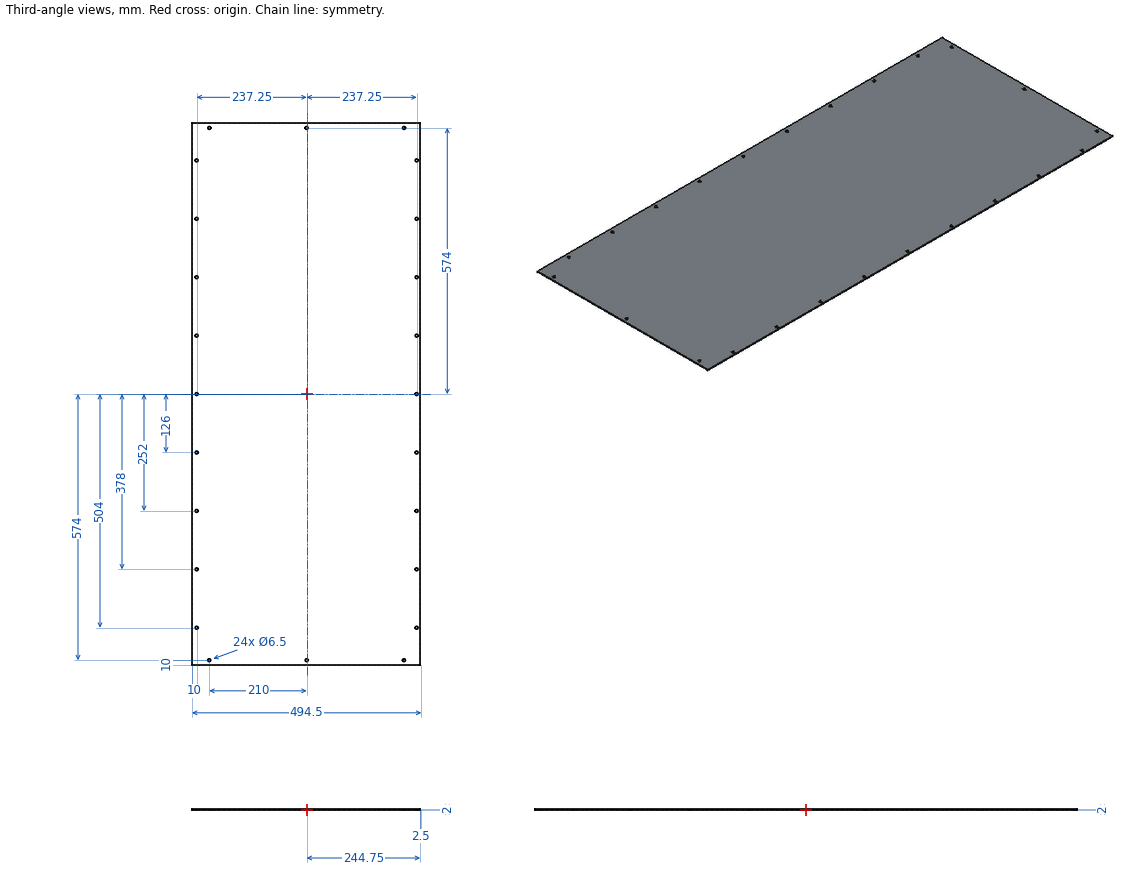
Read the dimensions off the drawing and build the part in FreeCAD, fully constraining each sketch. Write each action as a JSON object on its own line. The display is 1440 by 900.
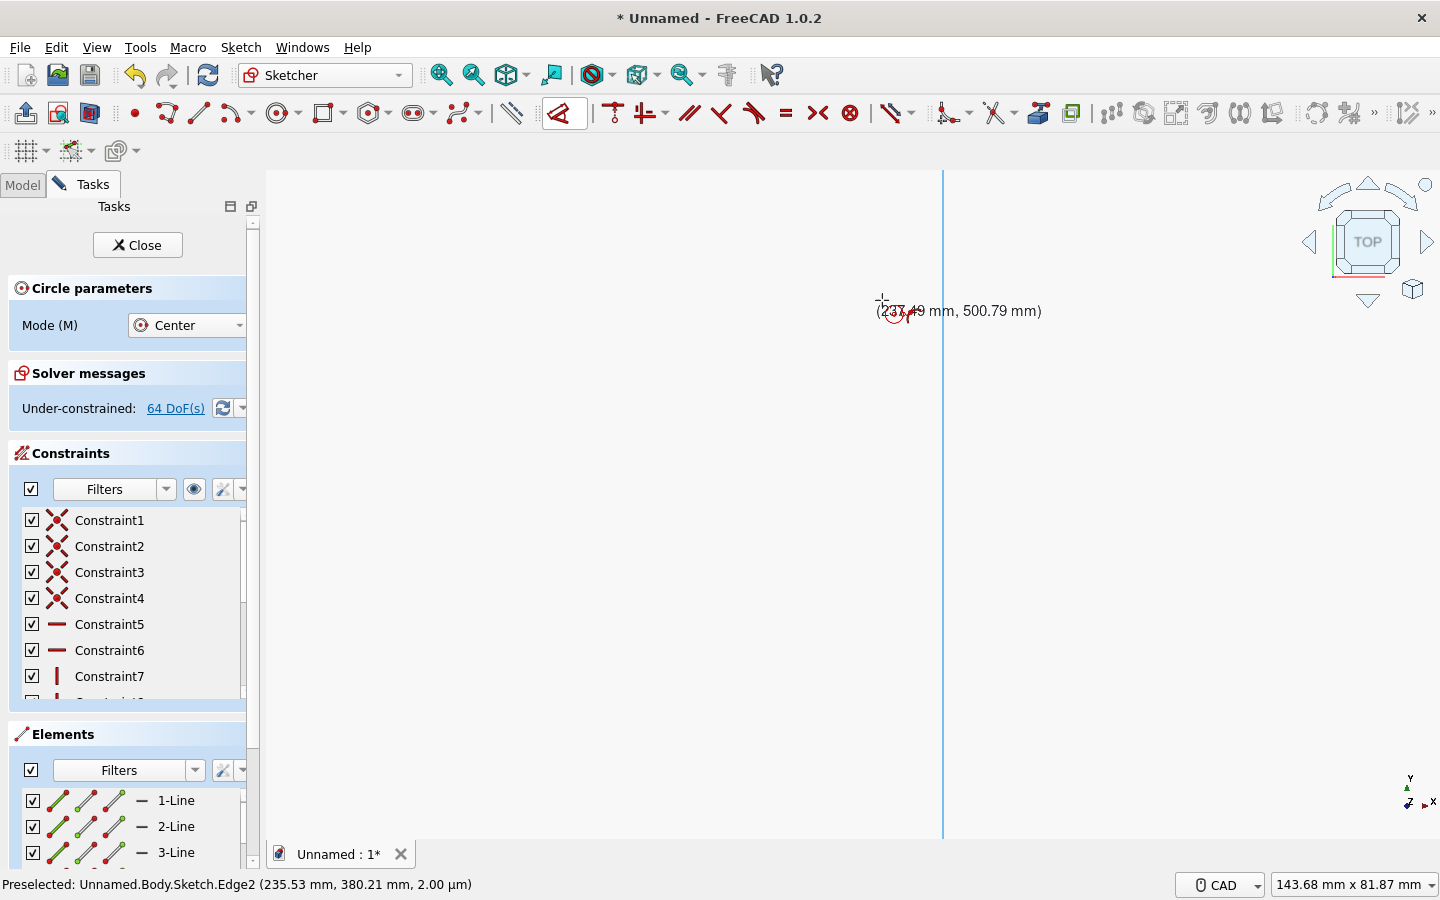
{"action": "scroll", "coordinate": [882, 300], "scroll_direction": "down", "scroll_amount": 15}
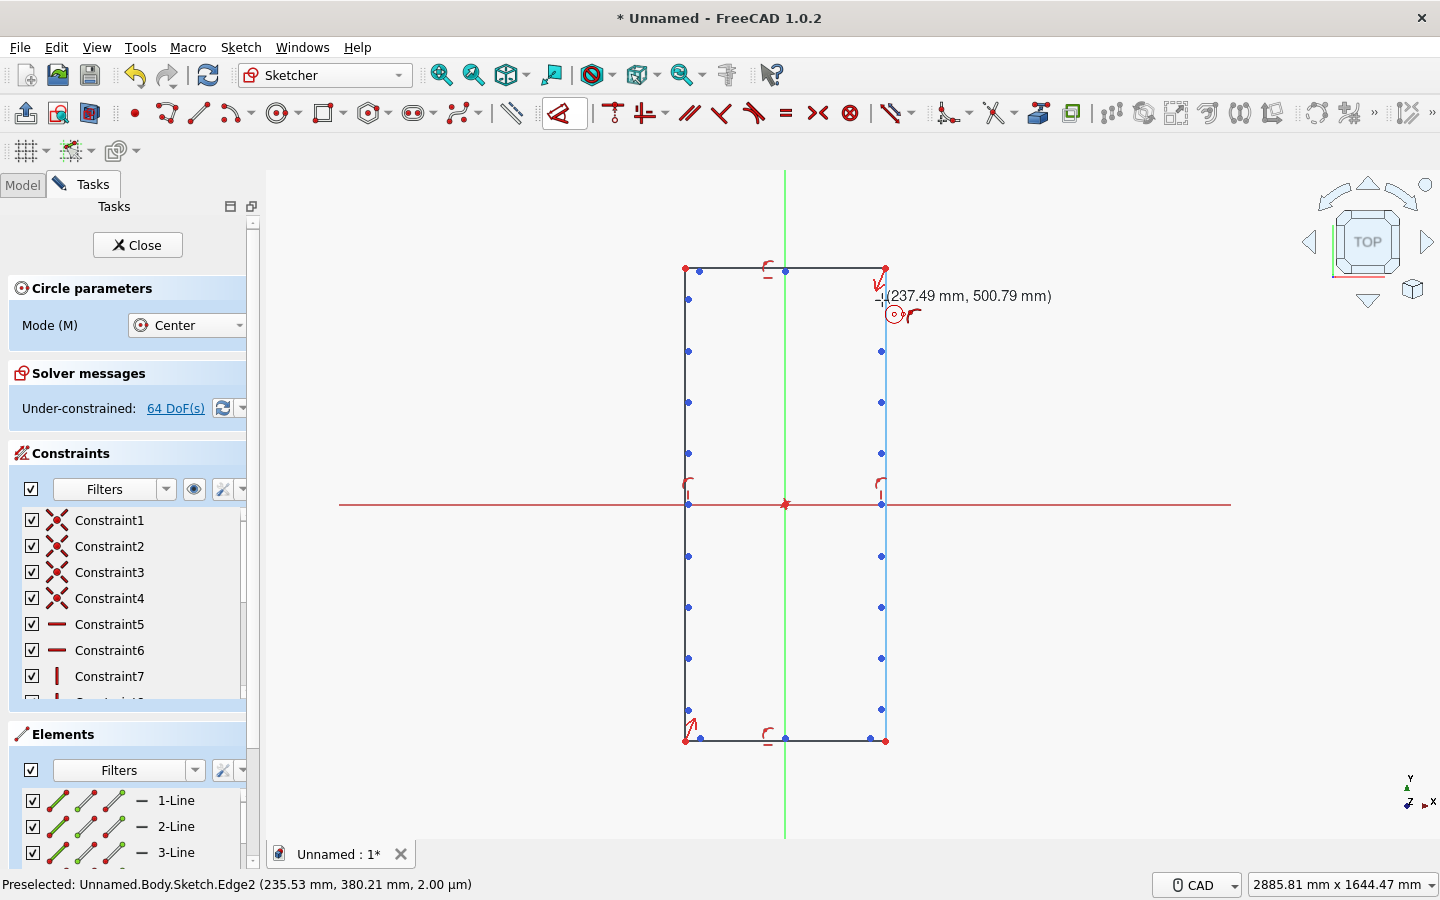
{"action": "scroll", "coordinate": [882, 300], "scroll_direction": "up", "scroll_amount": 7}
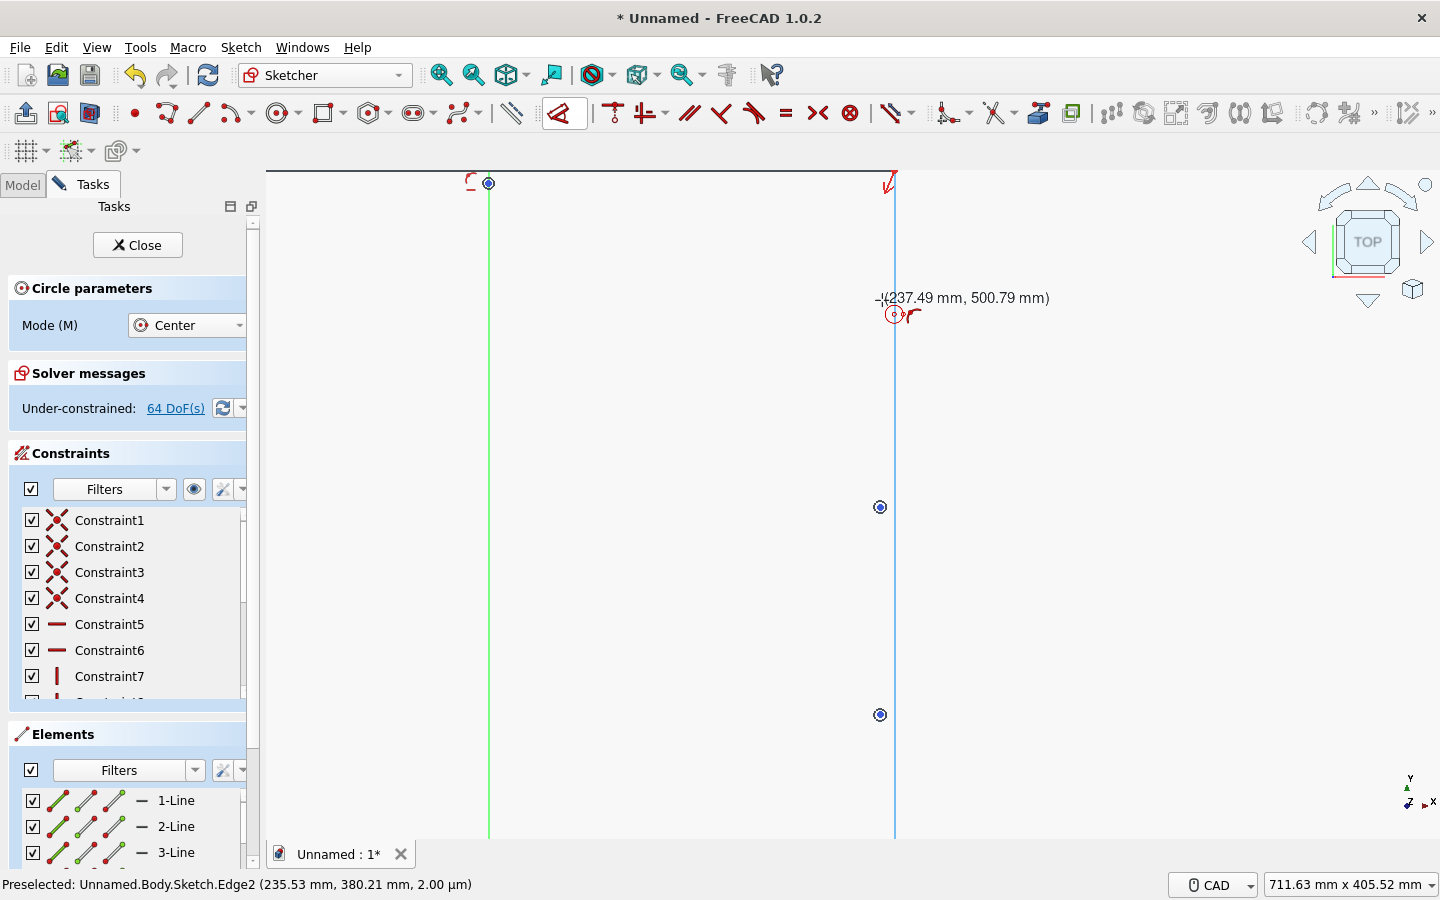
{"action": "left_click", "coordinate": [880, 298]}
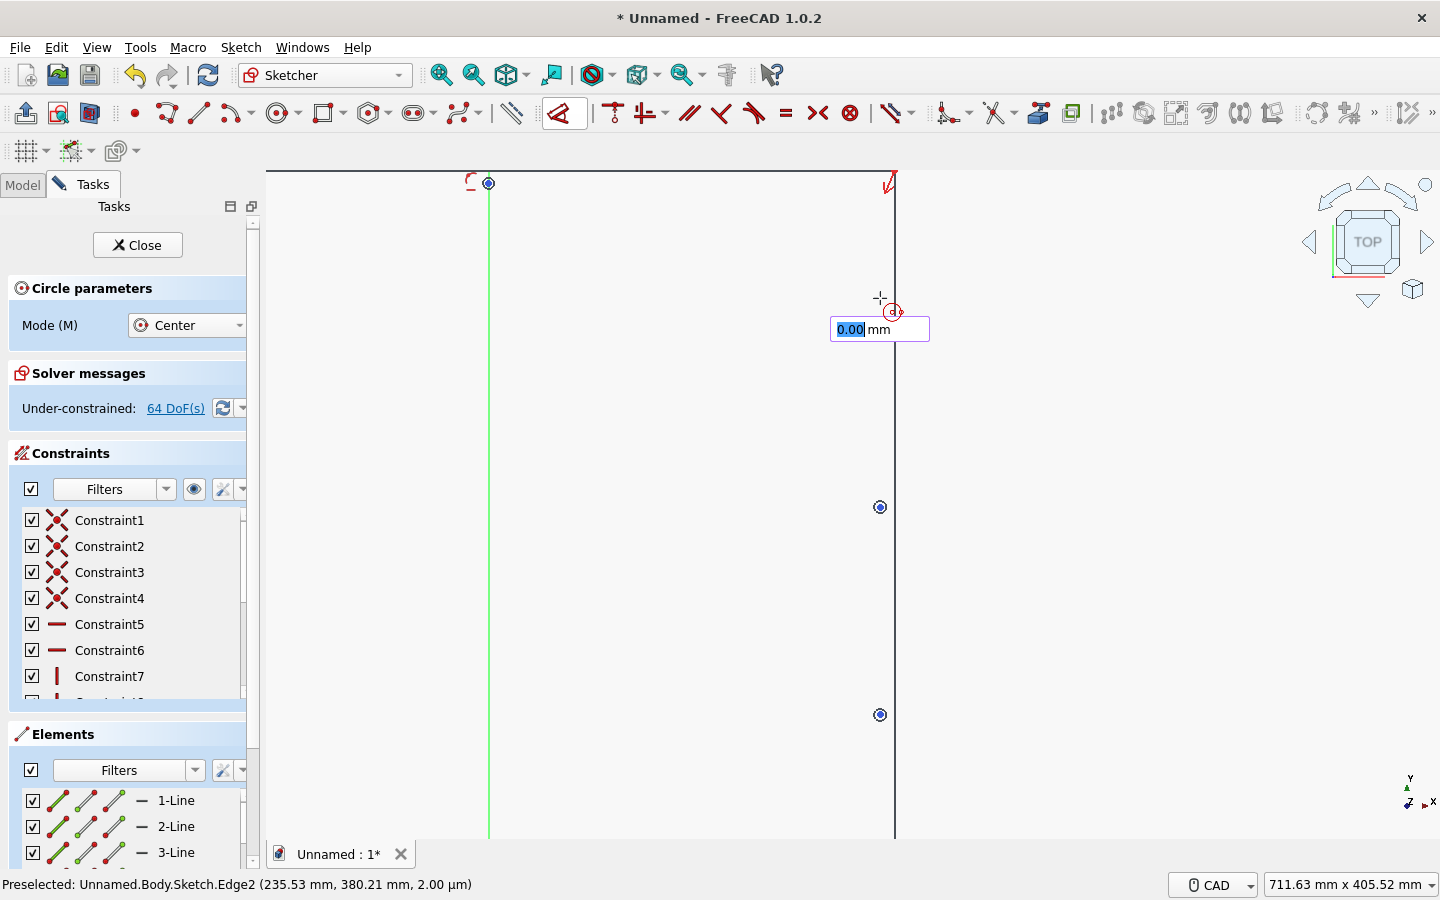
{"action": "scroll", "coordinate": [876, 294], "scroll_direction": "up", "scroll_amount": 6}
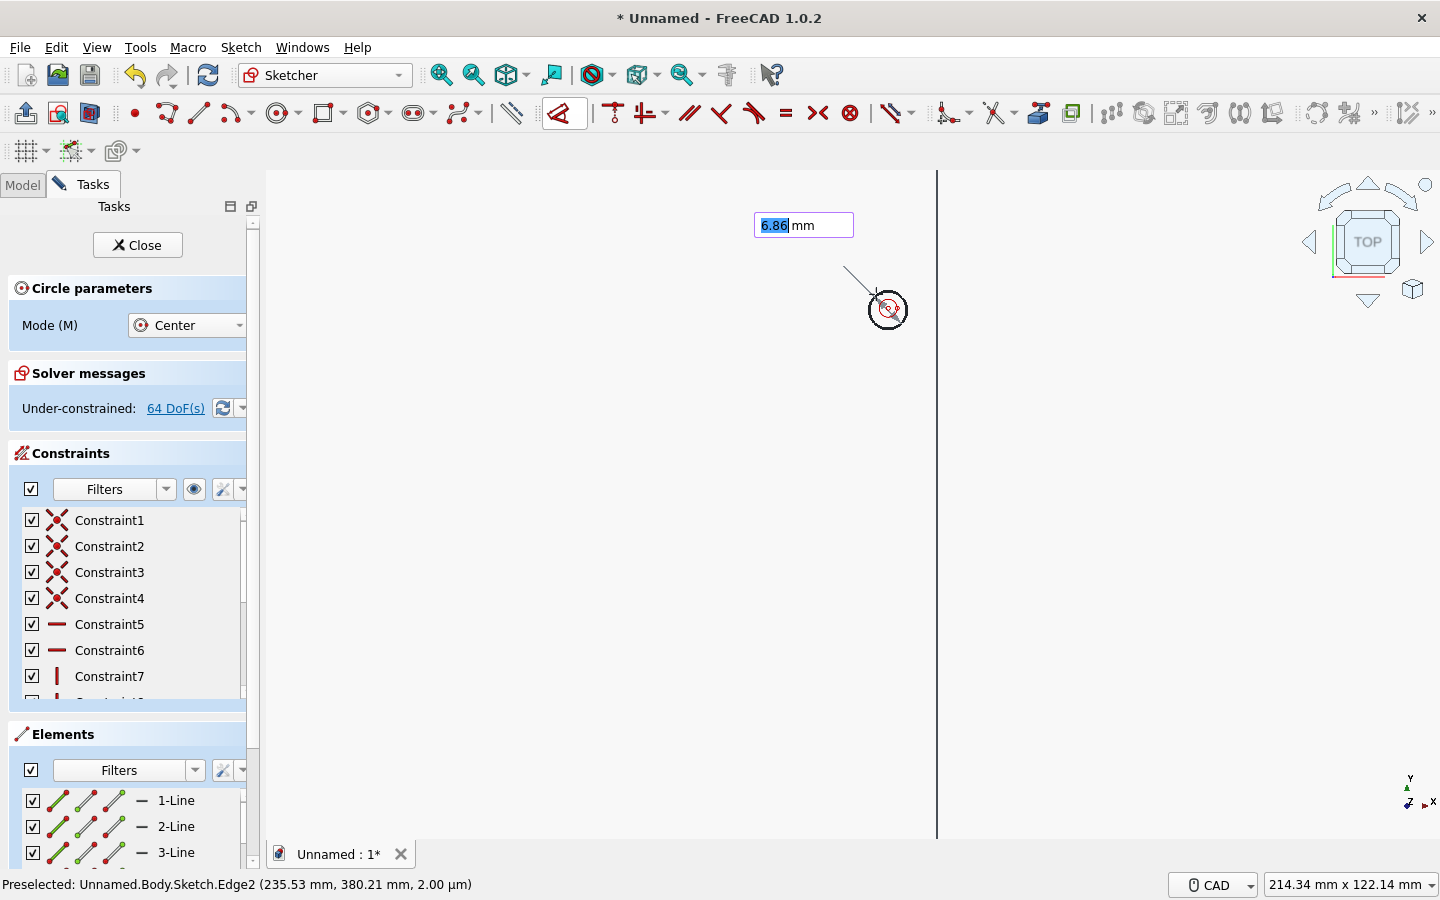
{"action": "left_click", "coordinate": [875, 295]}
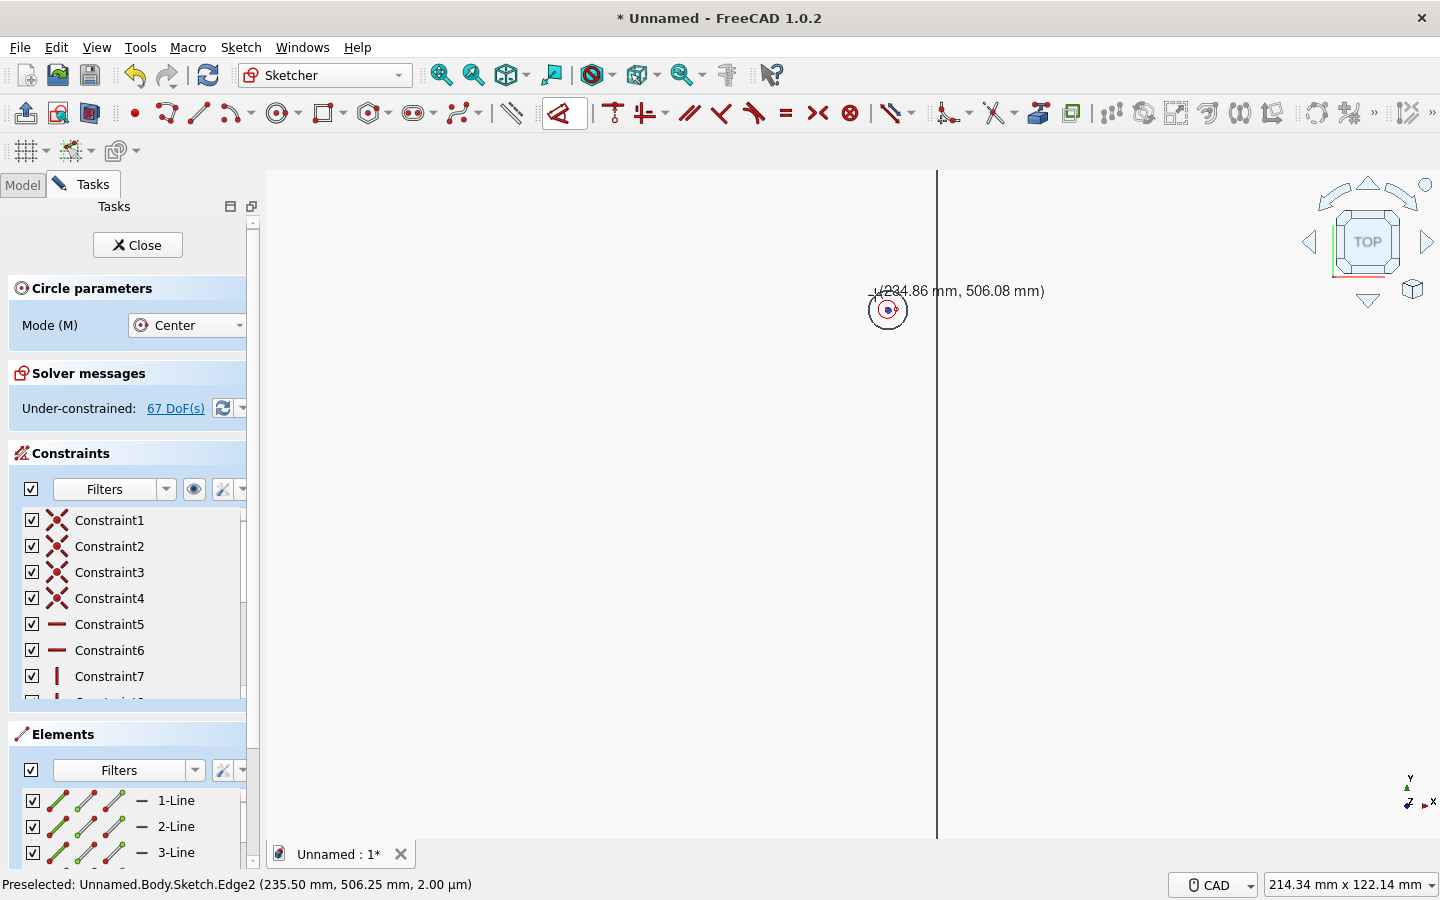
{"action": "scroll", "coordinate": [880, 299], "scroll_direction": "down", "scroll_amount": 13}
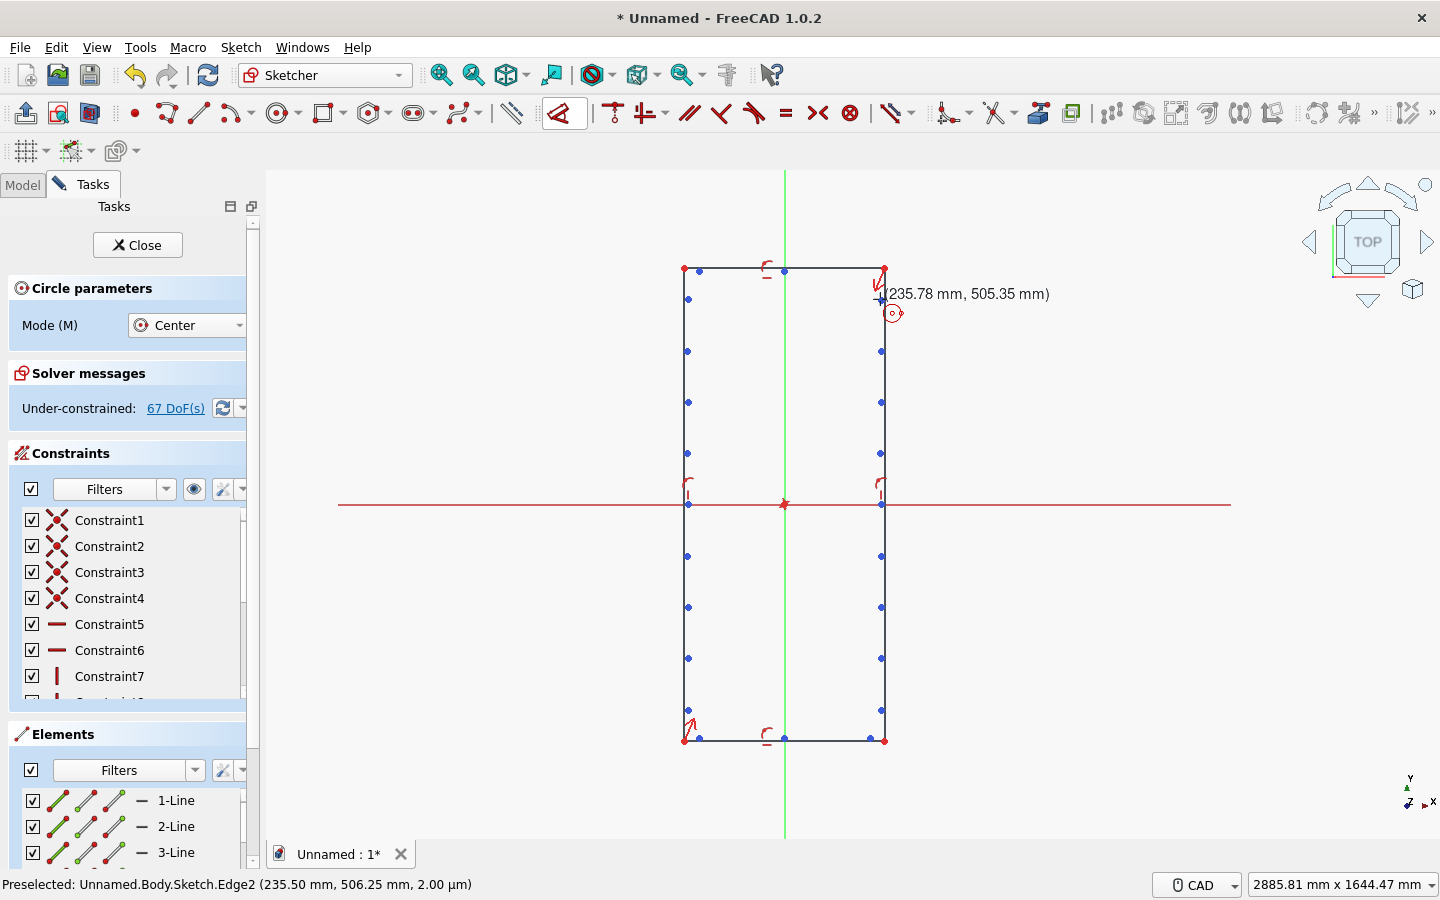
{"action": "scroll", "coordinate": [870, 271], "scroll_direction": "up", "scroll_amount": 15}